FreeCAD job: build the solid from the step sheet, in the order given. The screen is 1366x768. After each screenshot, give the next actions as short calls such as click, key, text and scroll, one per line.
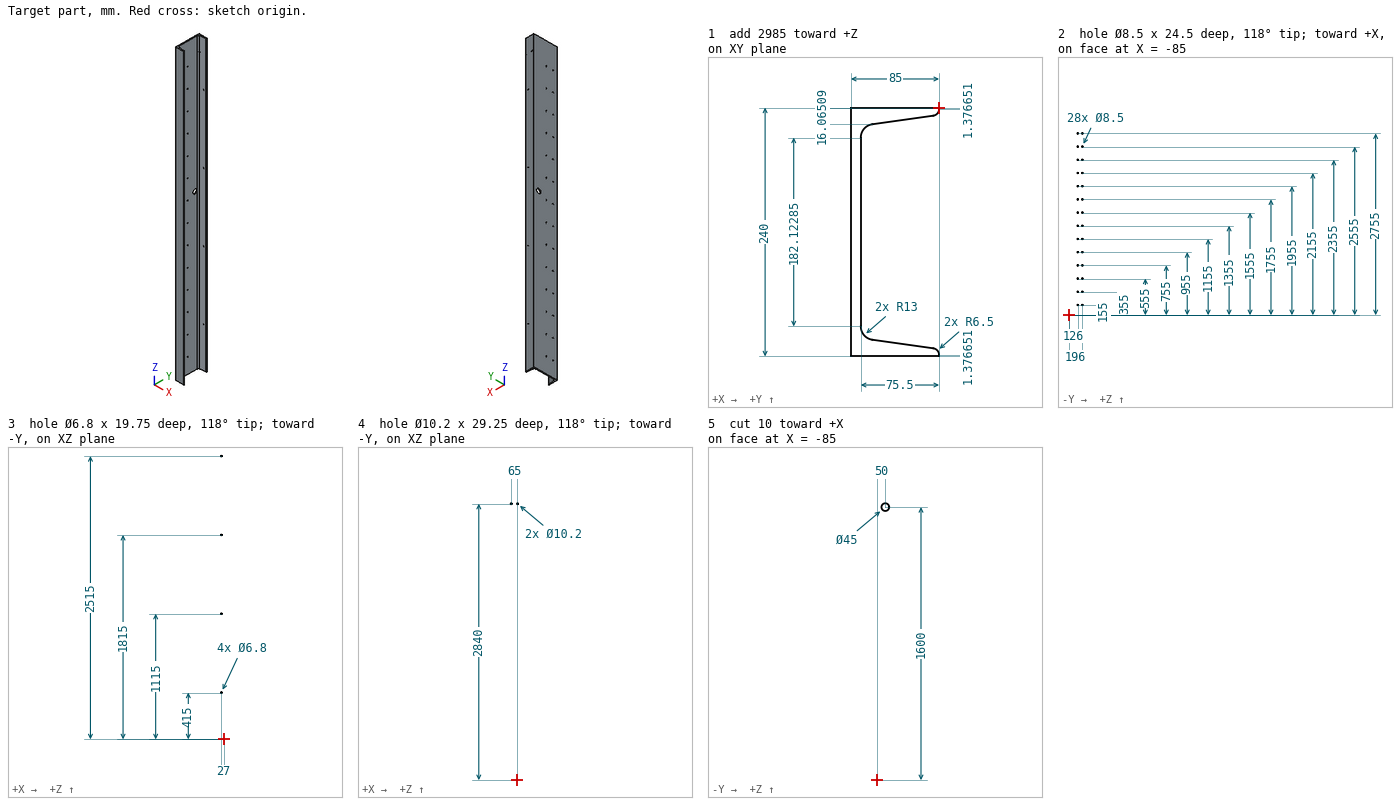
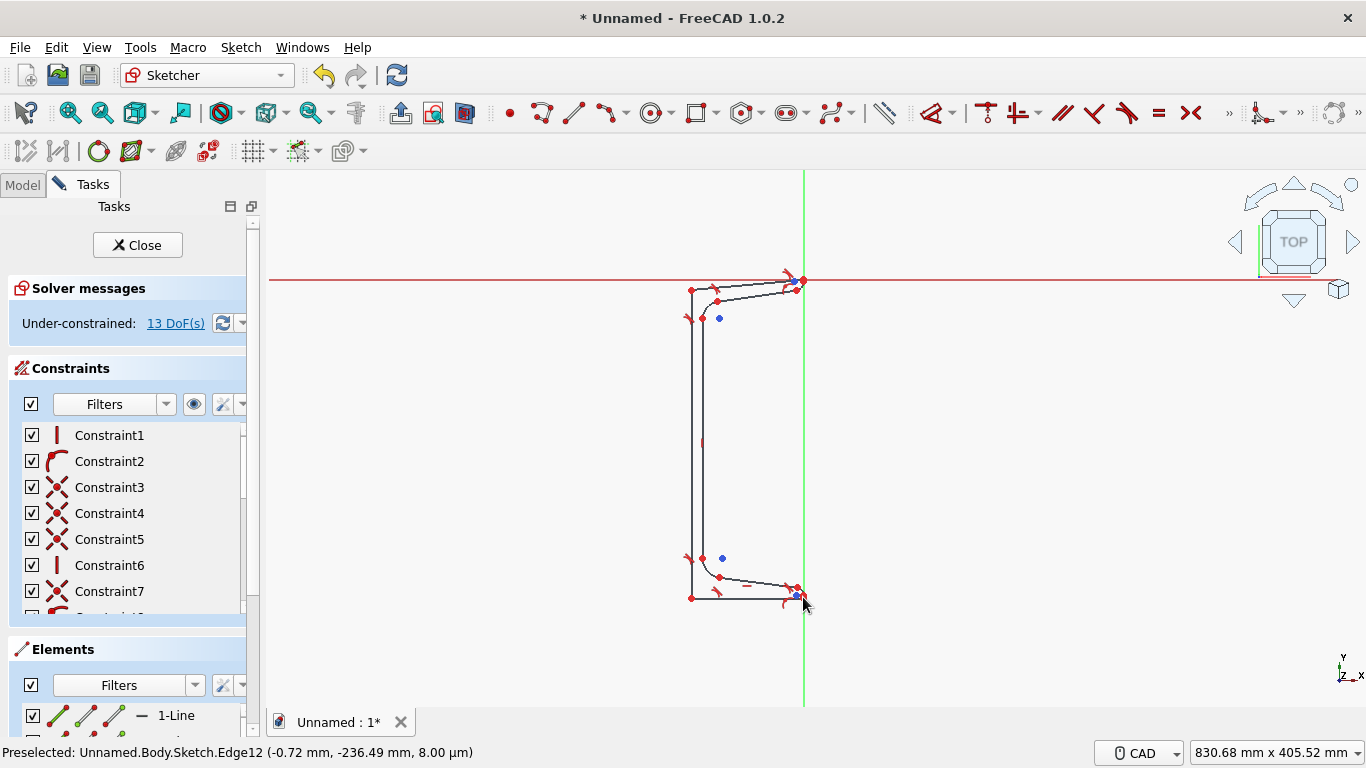
scroll(770, 283, up, 8)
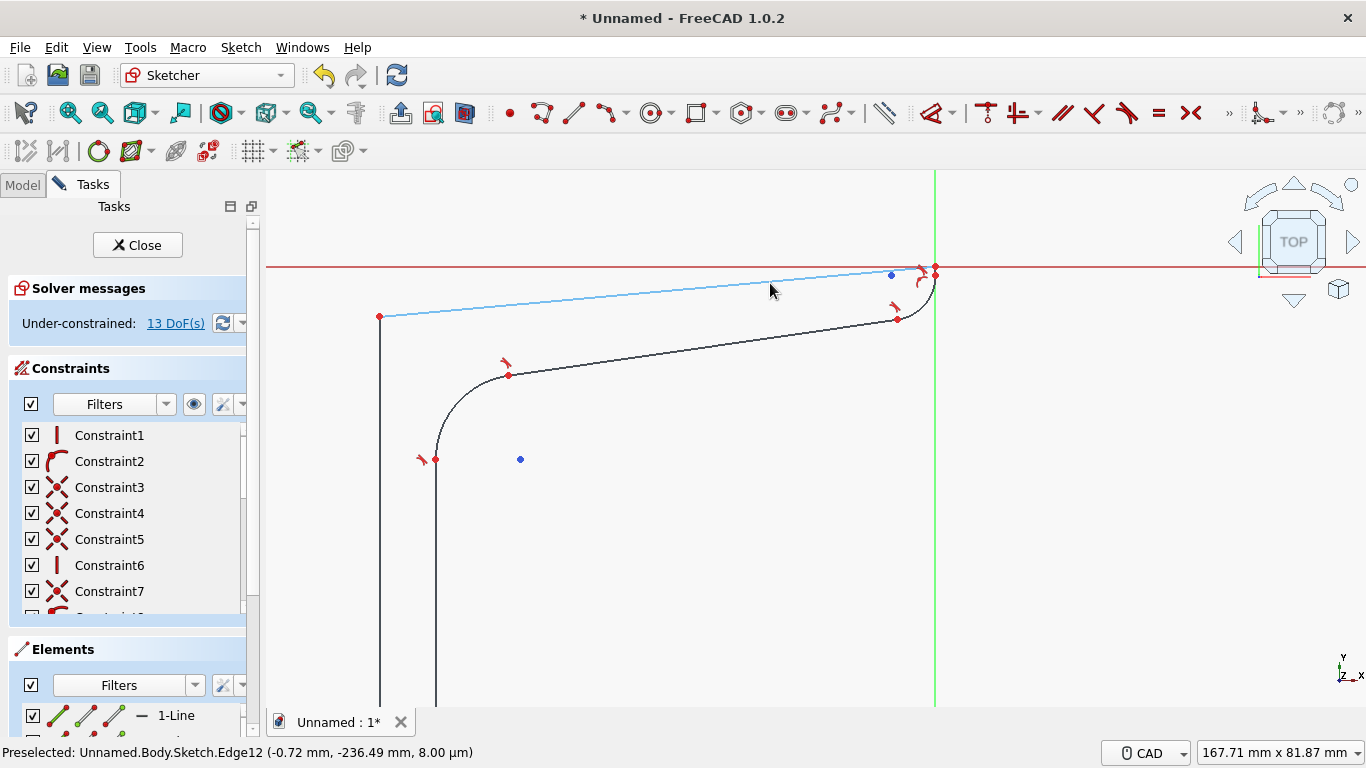
click(769, 282)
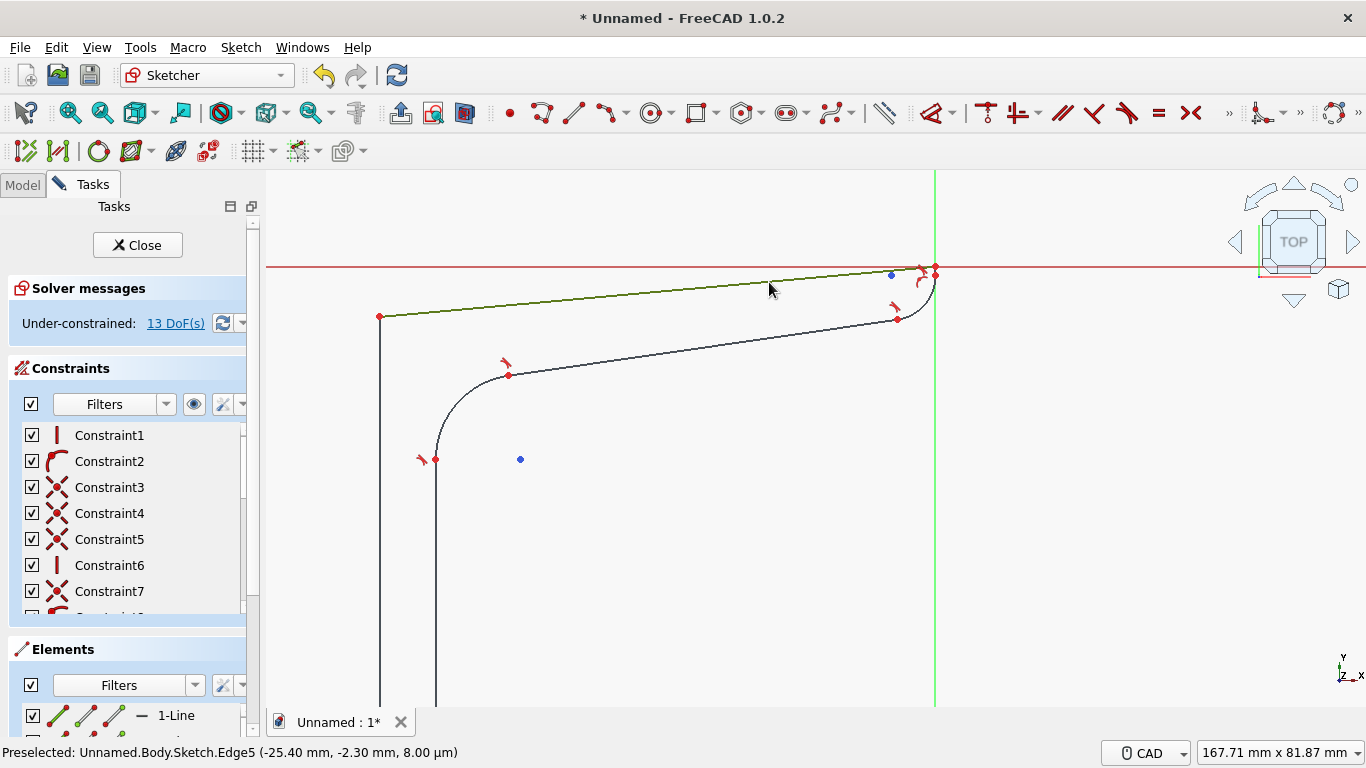
click(1040, 114)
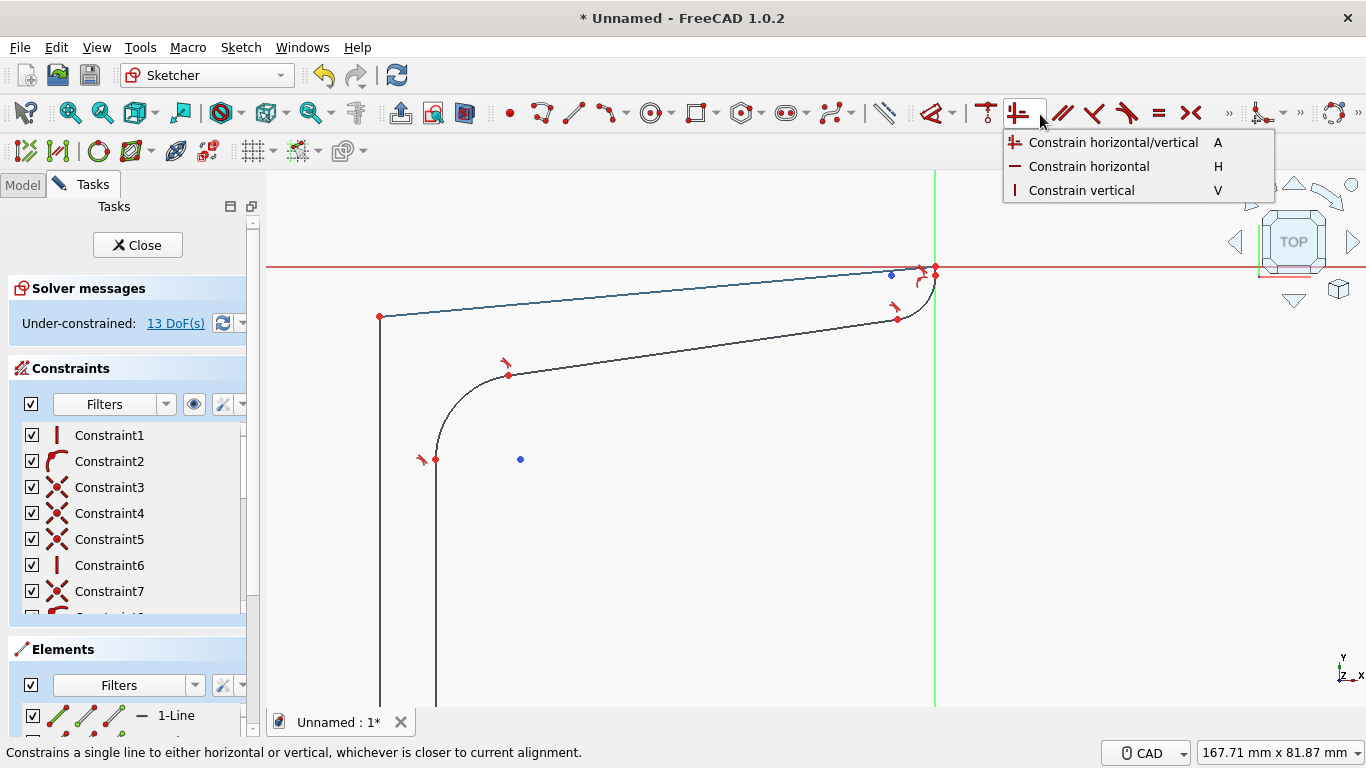
click(1139, 166)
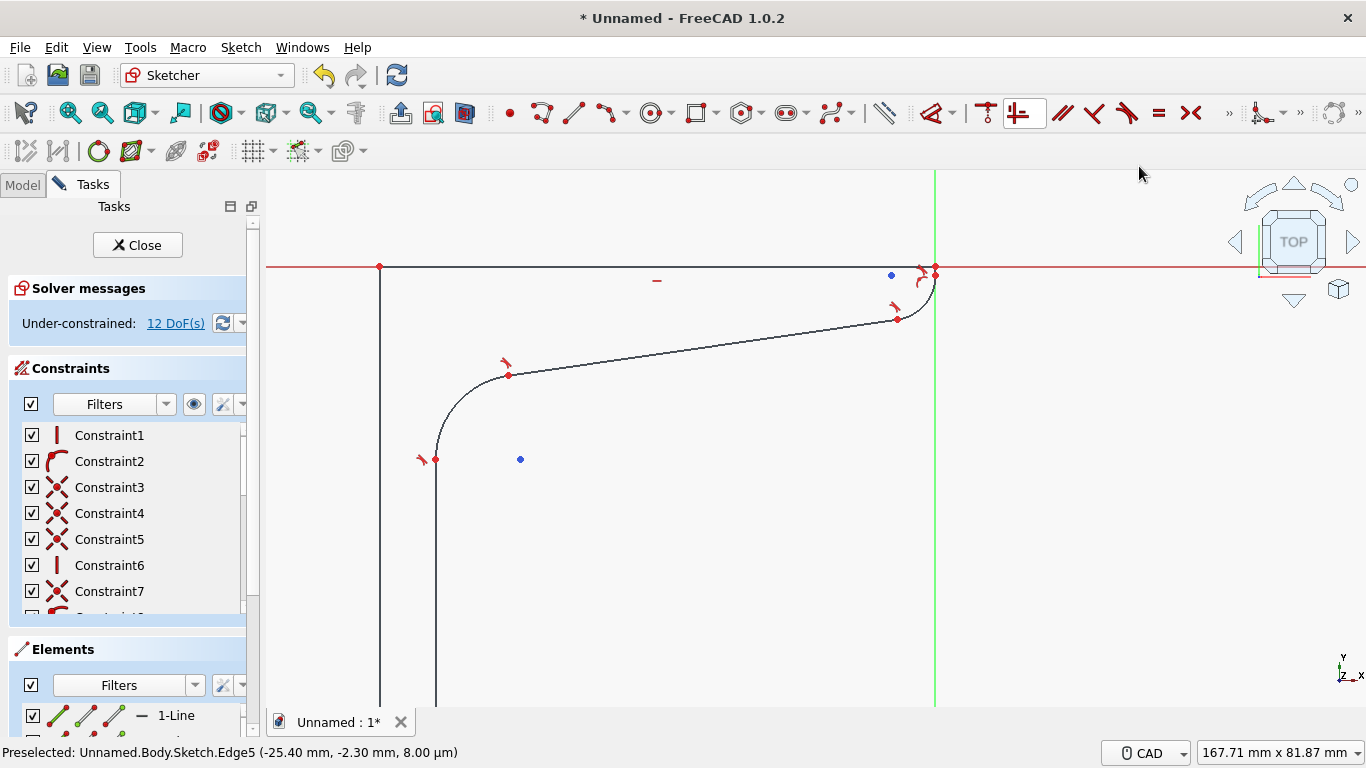
scroll(770, 283, down, 8)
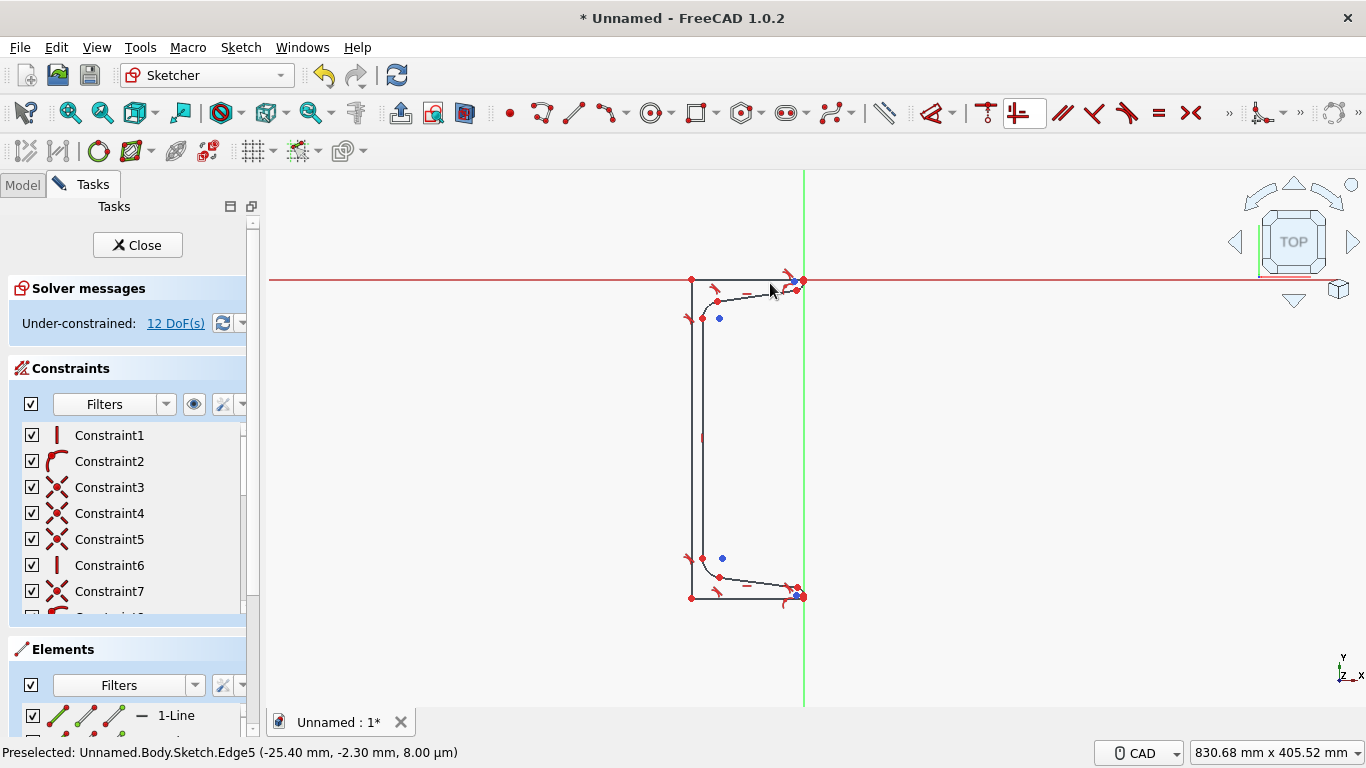
scroll(705, 567, up, 3)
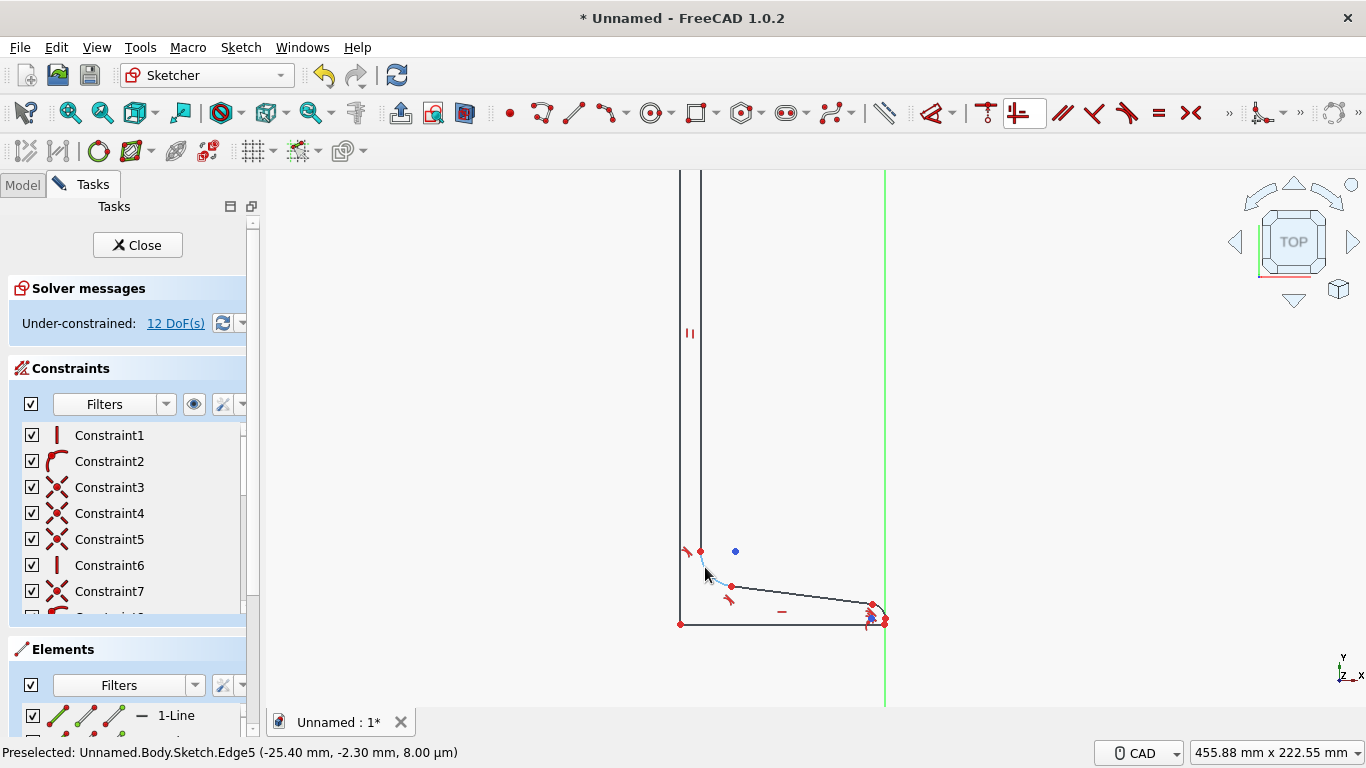
click(704, 566)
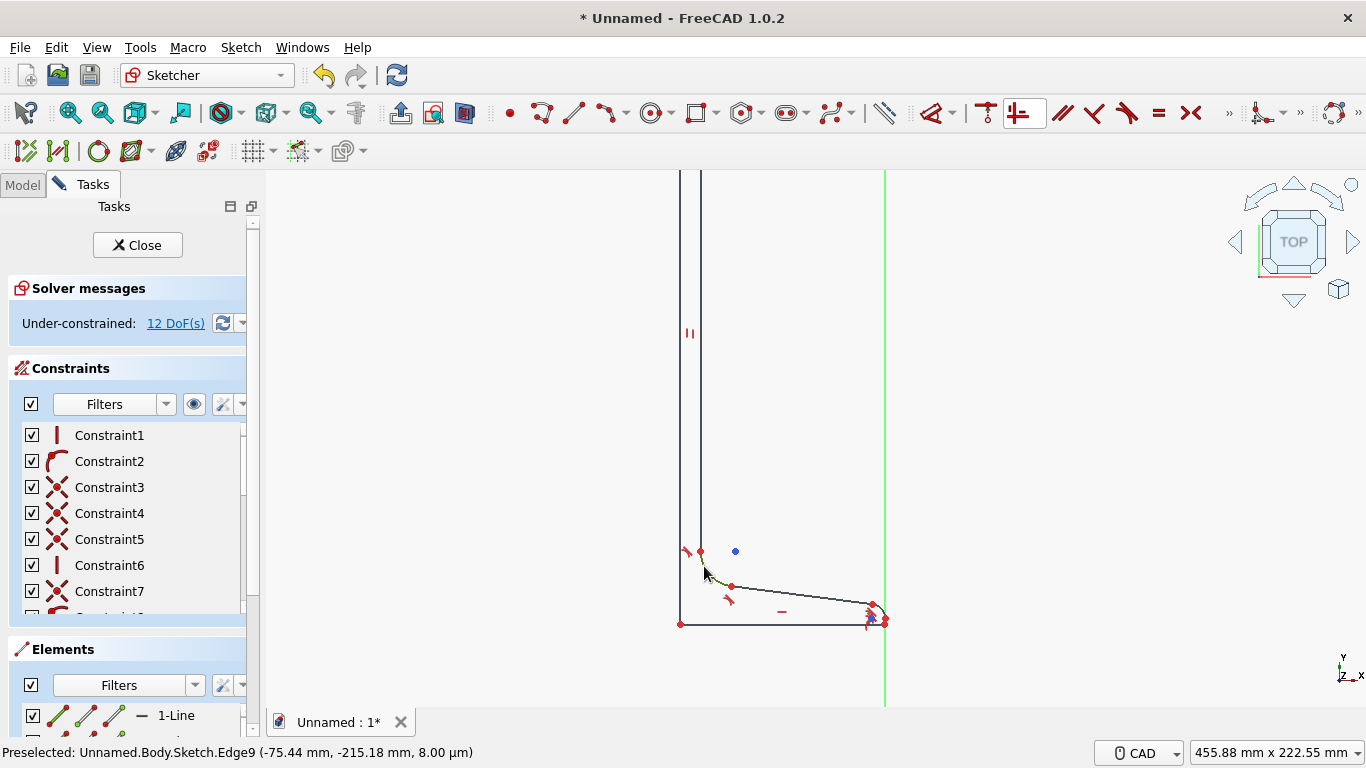
scroll(705, 567, down, 3)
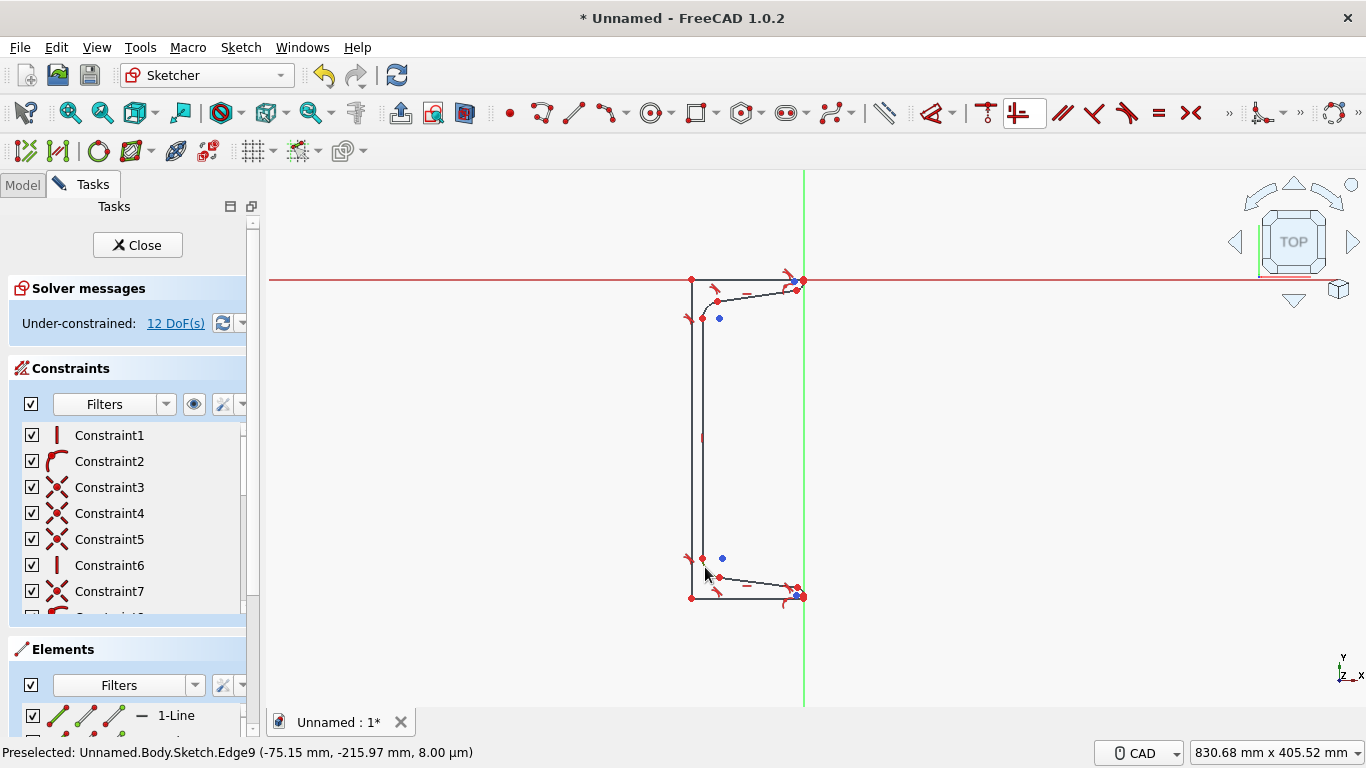
scroll(711, 304, up, 4)